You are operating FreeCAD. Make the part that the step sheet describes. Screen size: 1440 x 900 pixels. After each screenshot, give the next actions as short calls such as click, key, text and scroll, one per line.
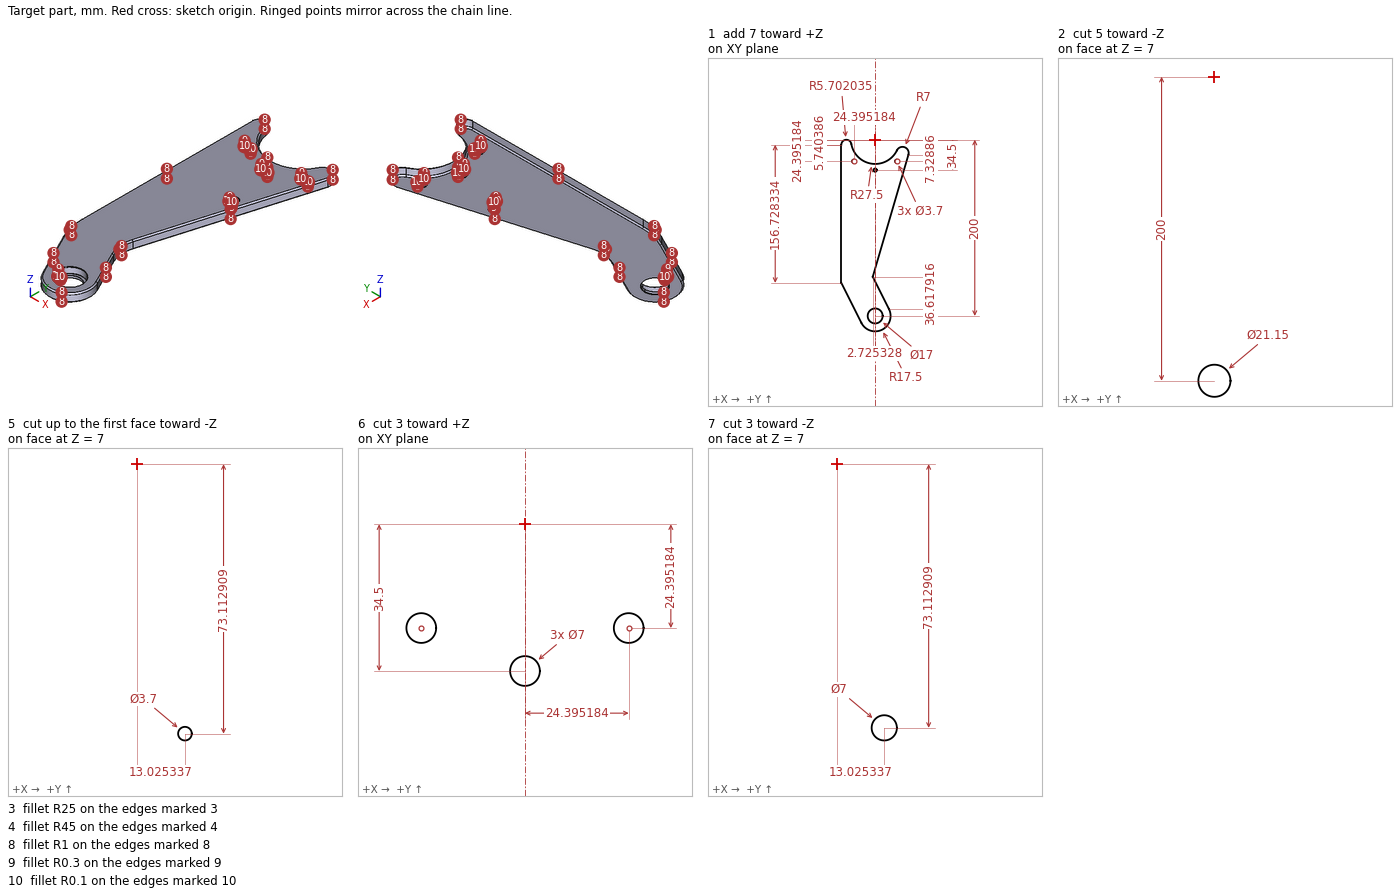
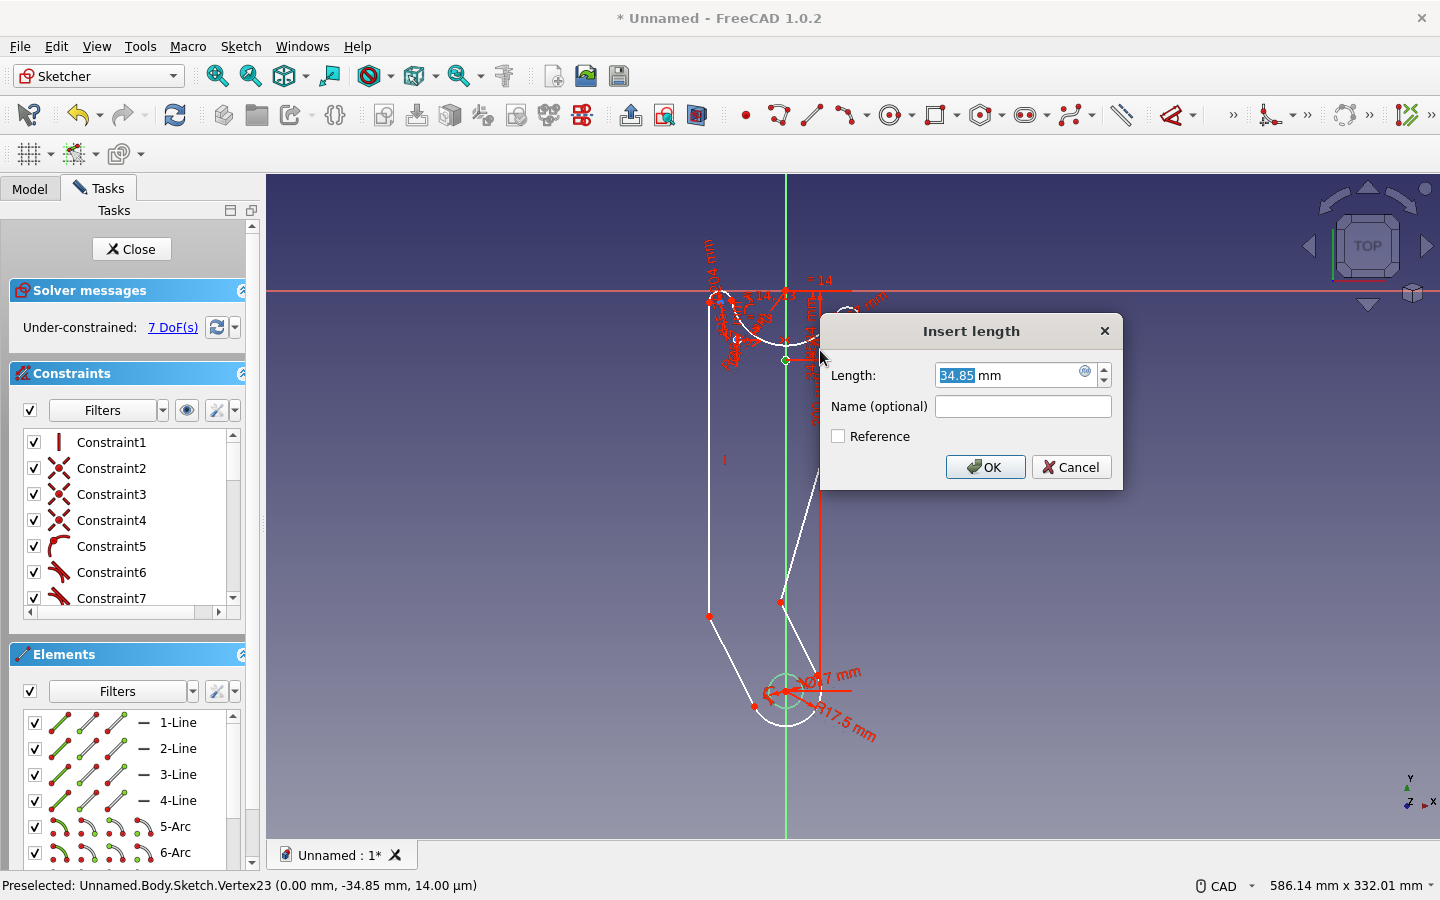
text(34.5)
key(Return)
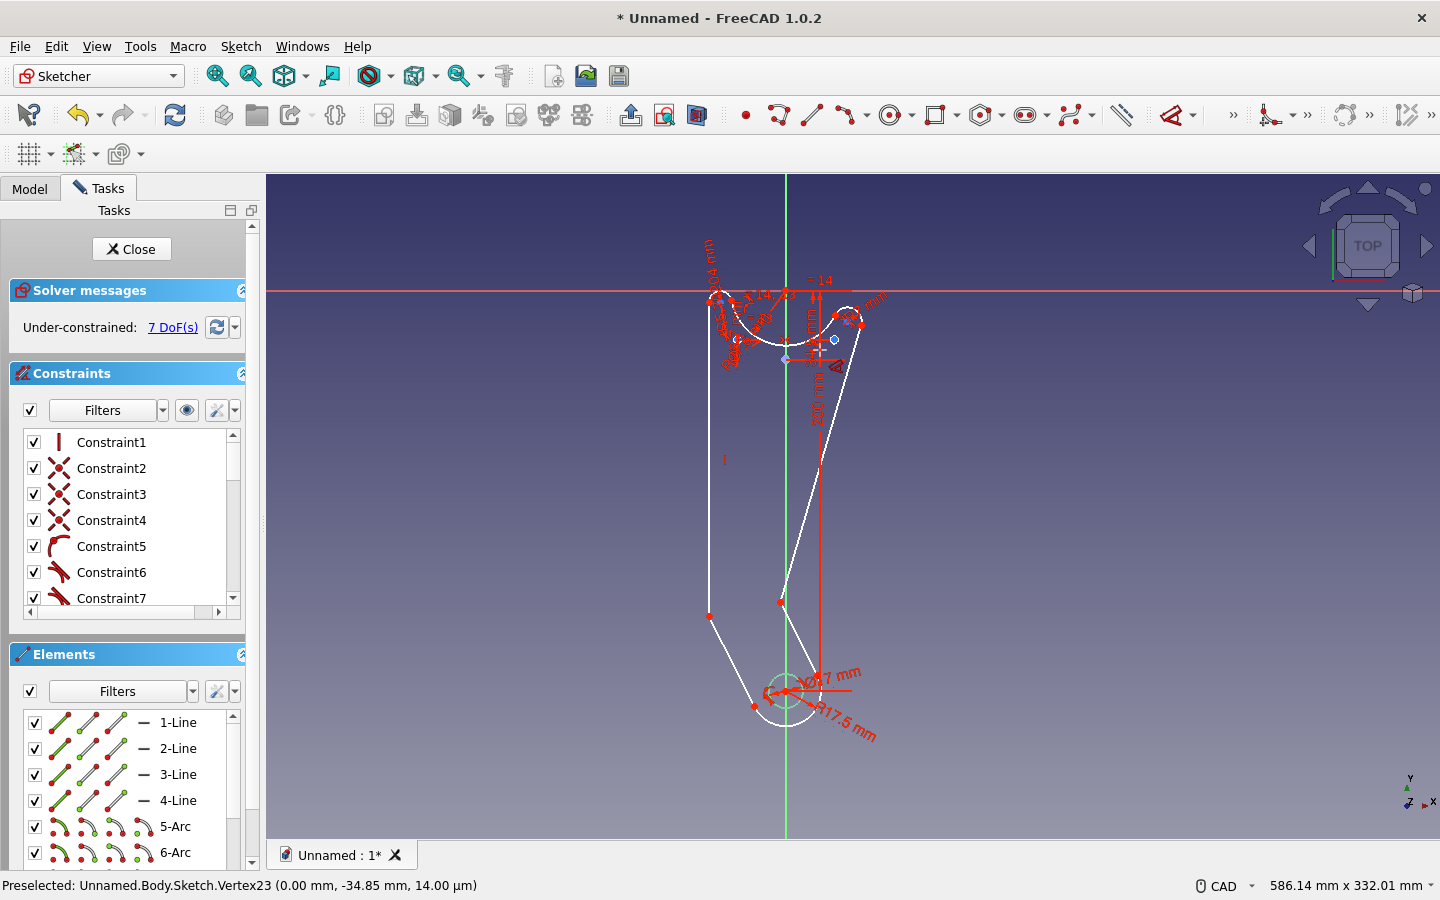
scroll(861, 325, up, 5)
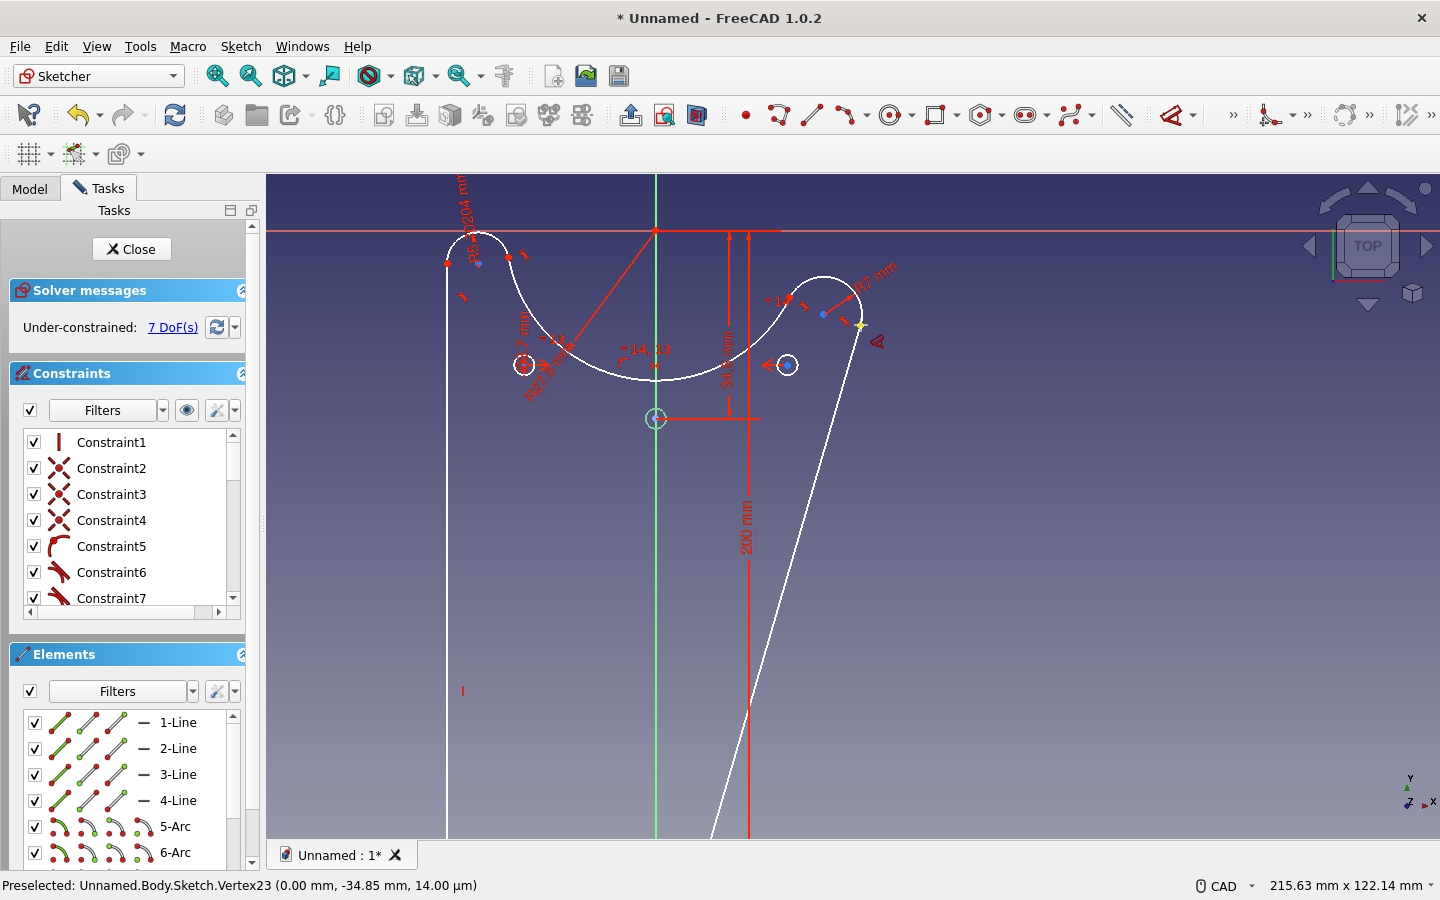
click(860, 326)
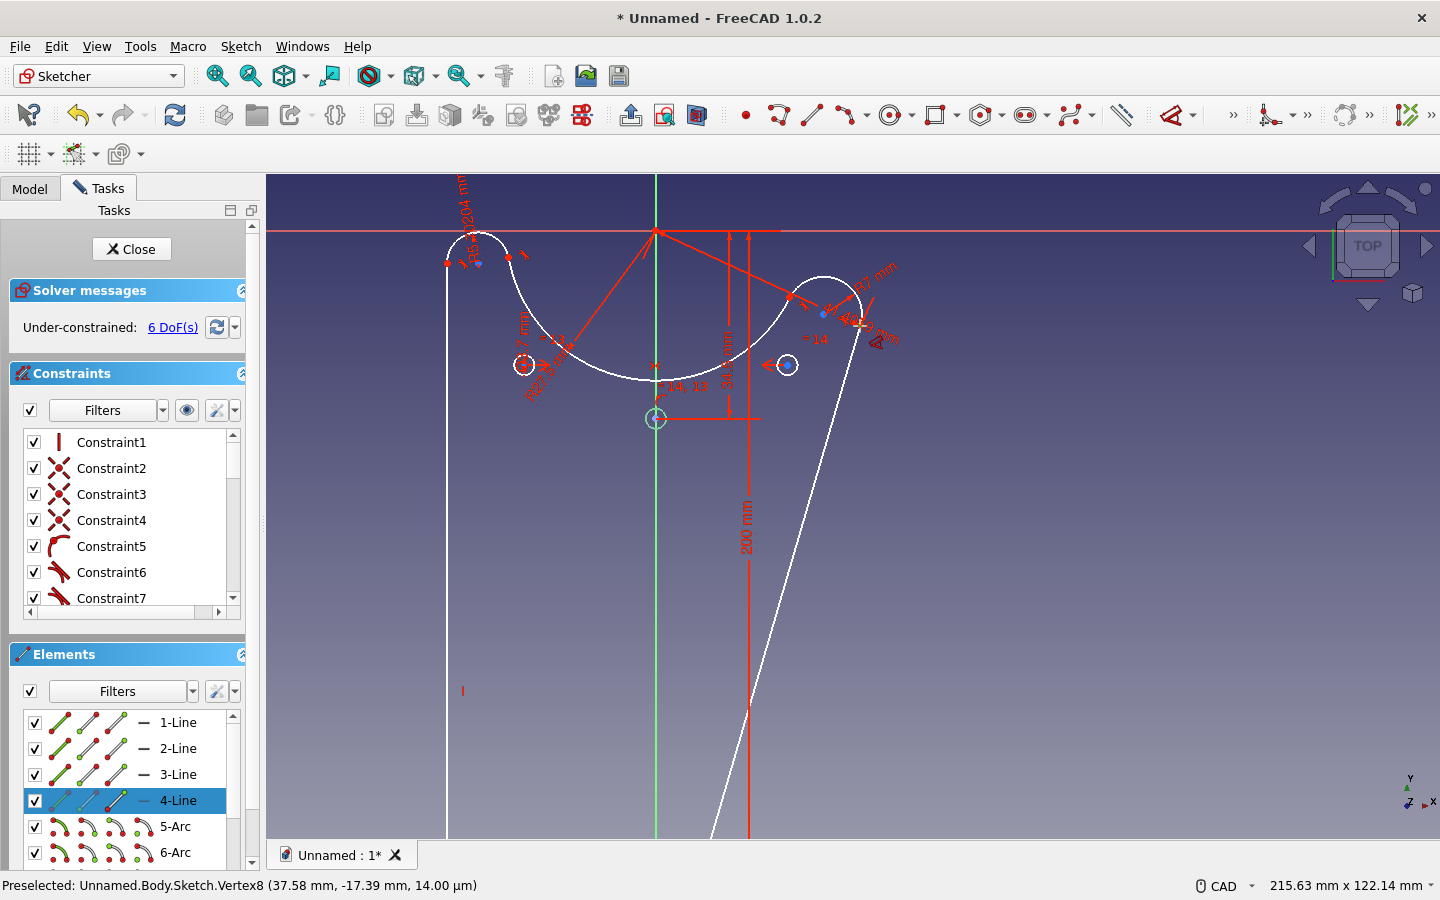
click(787, 365)
click(894, 345)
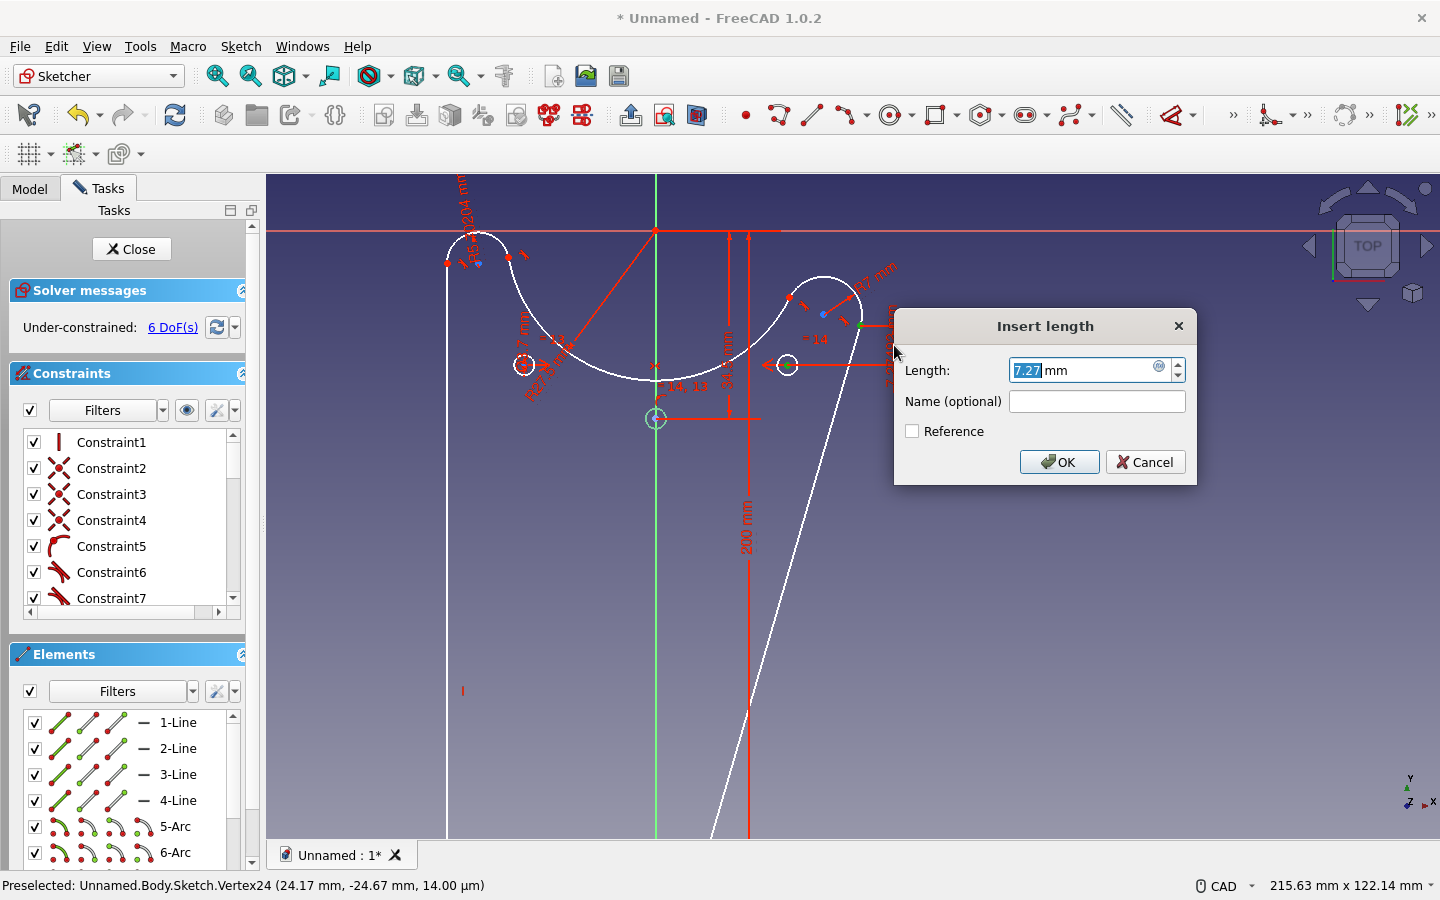
text(7.32886)
key(Return)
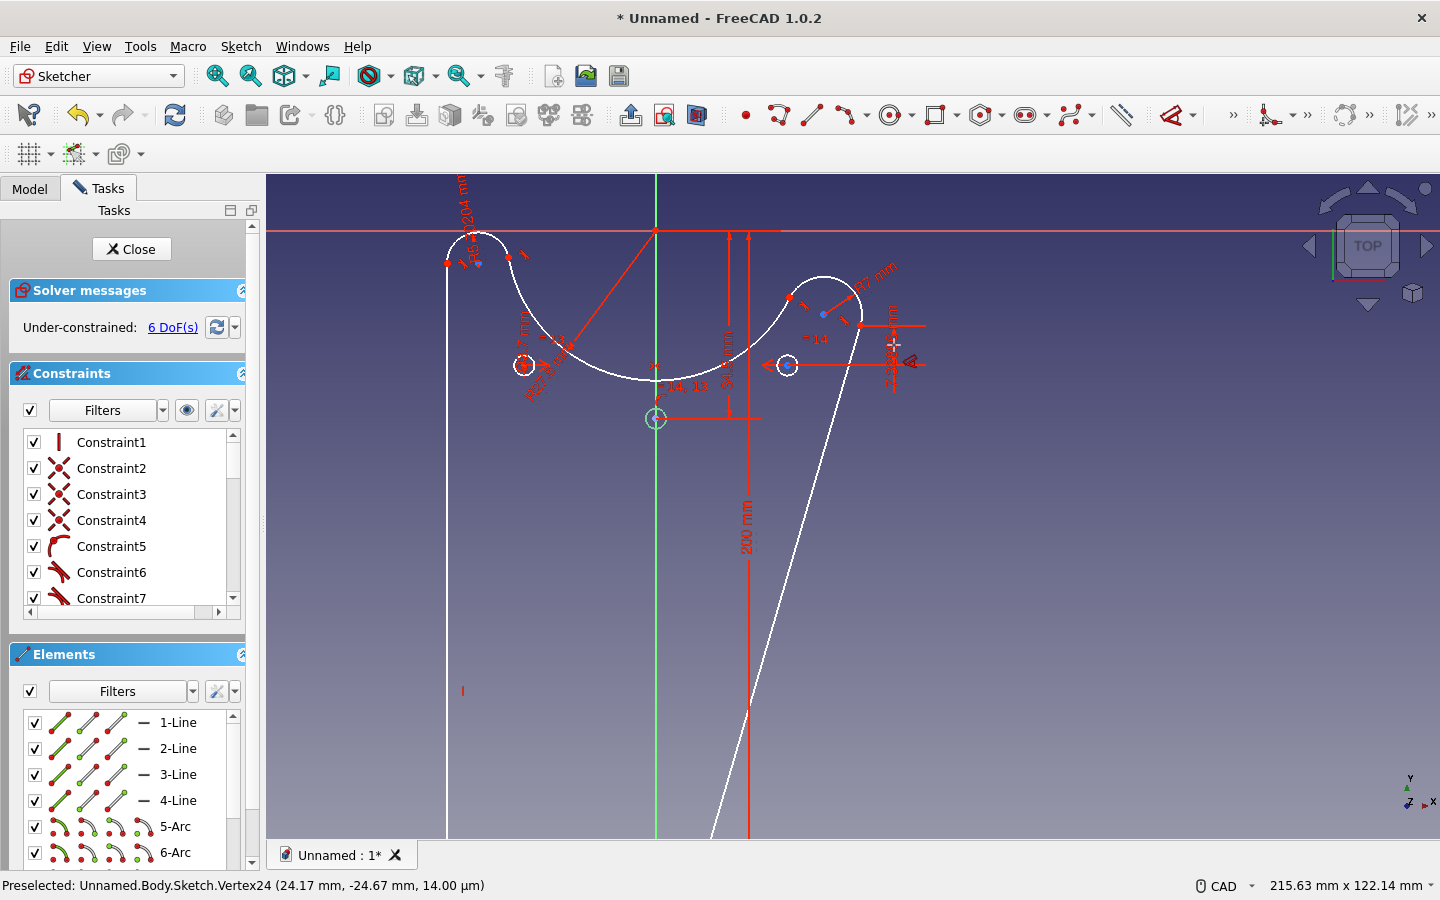
scroll(447, 263, up, 2)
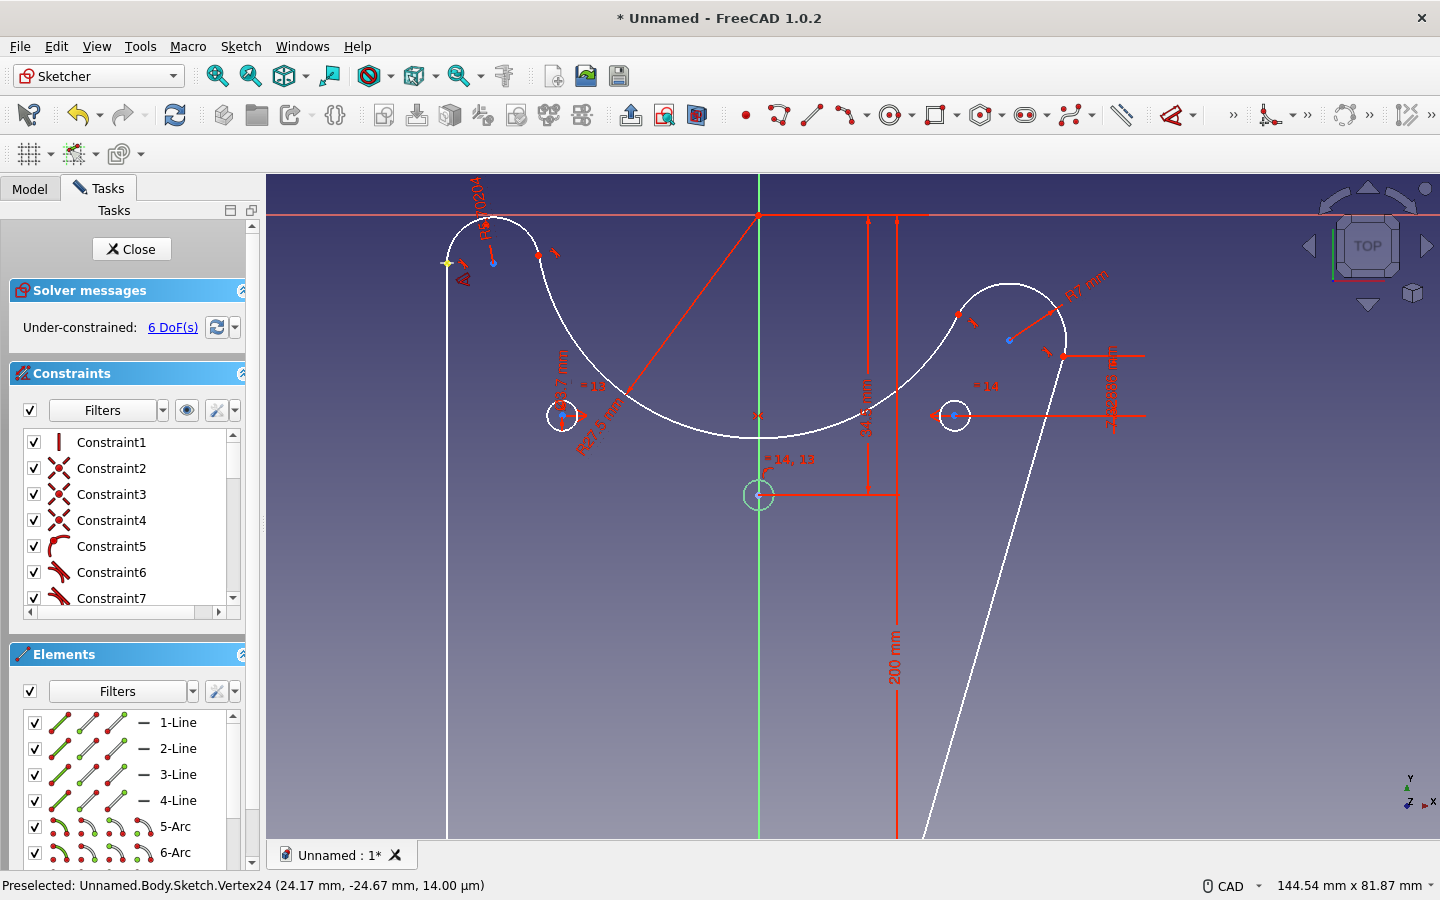
click(447, 264)
click(413, 239)